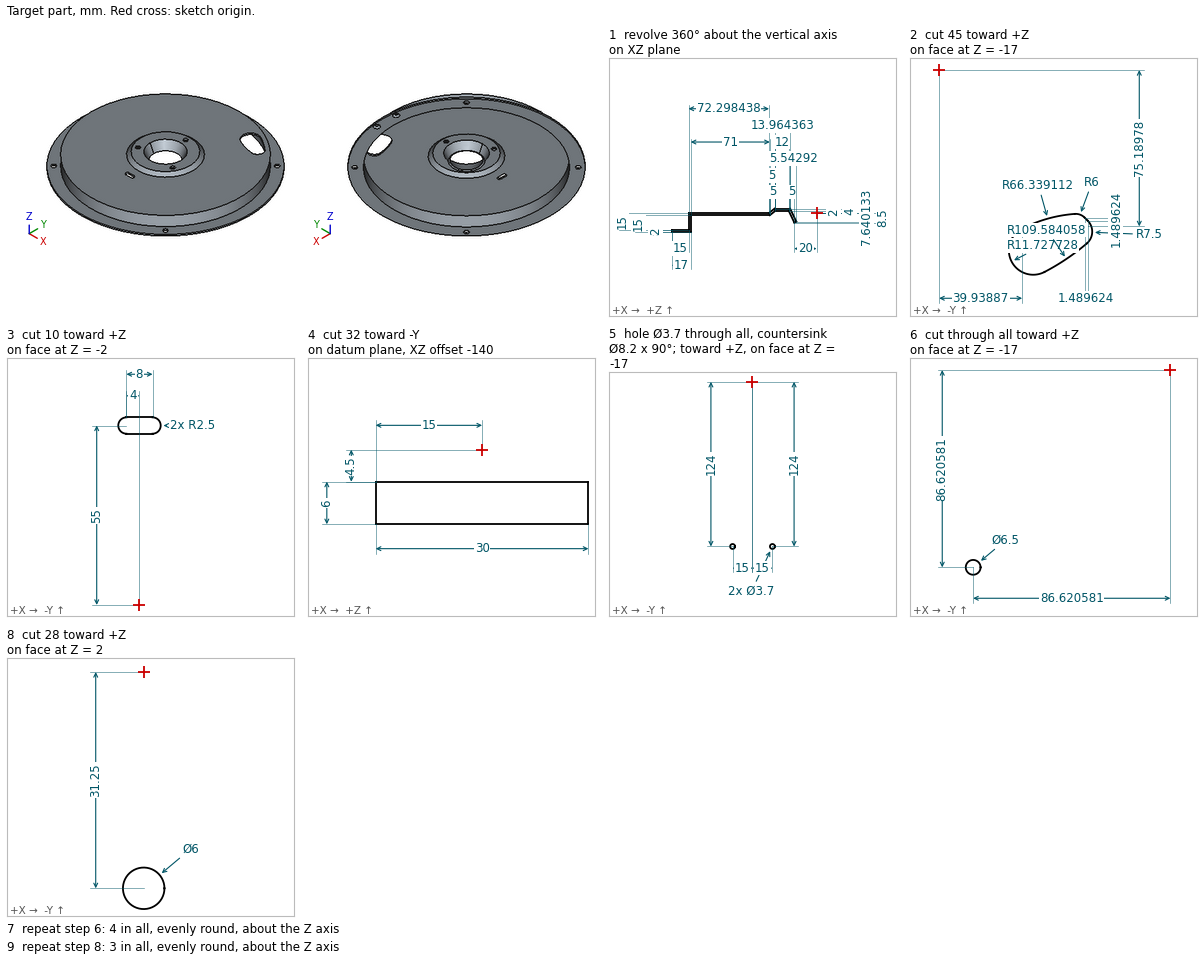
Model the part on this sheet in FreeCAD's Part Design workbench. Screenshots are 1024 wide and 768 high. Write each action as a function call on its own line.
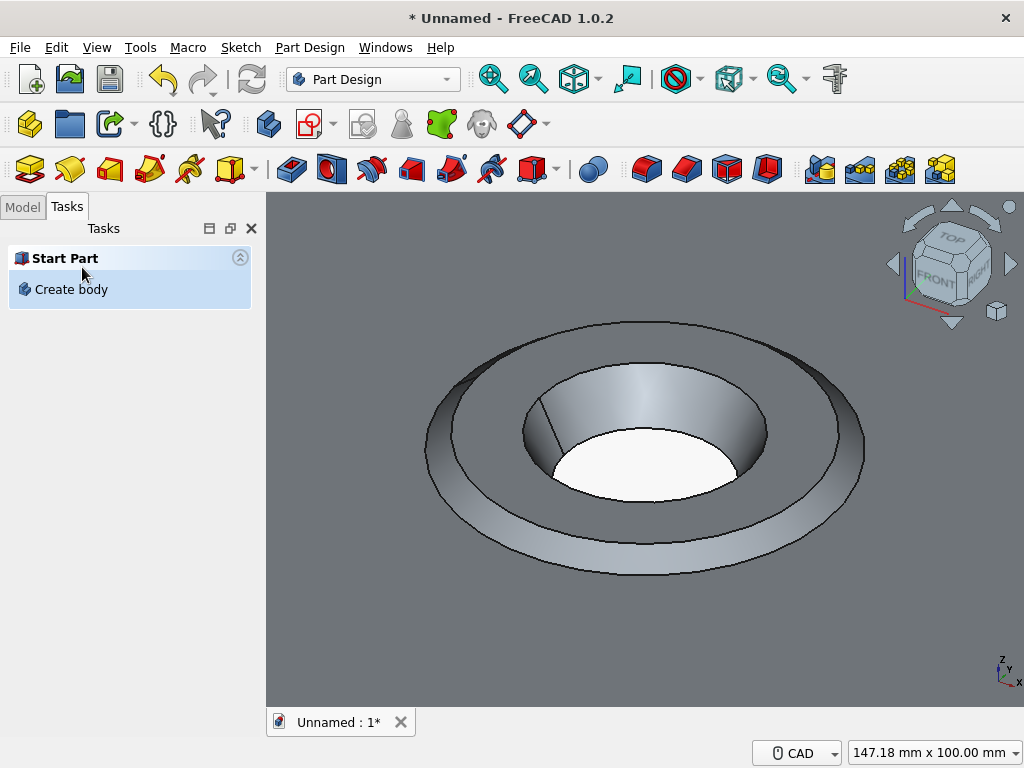
click(494, 80)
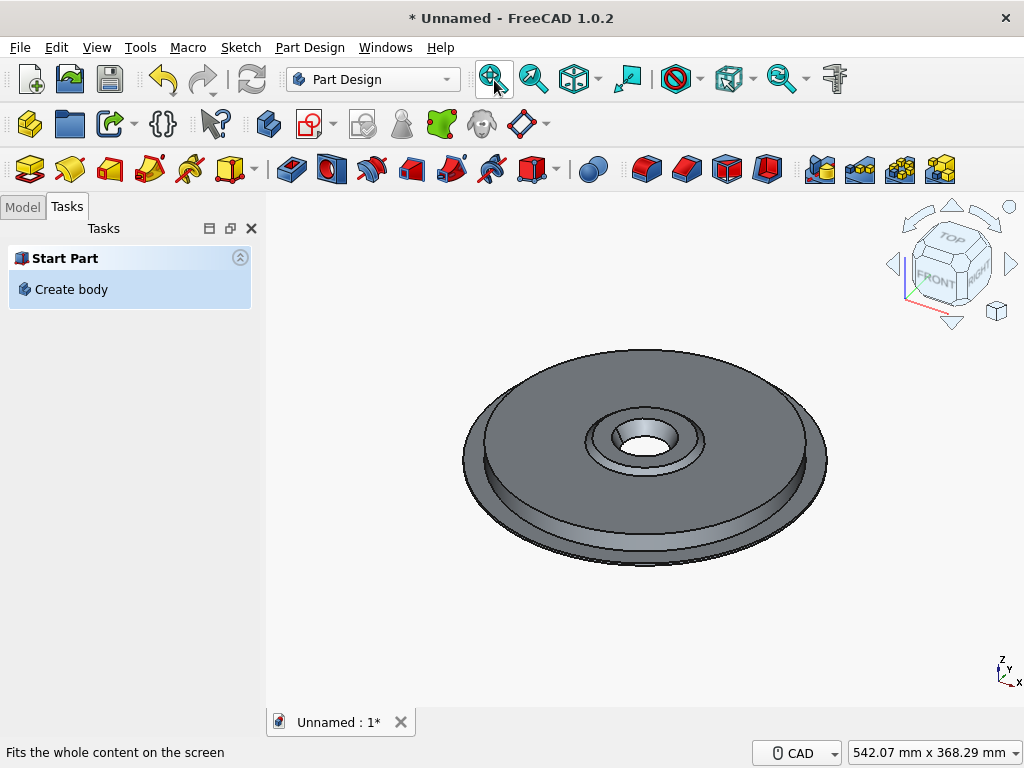
key(5)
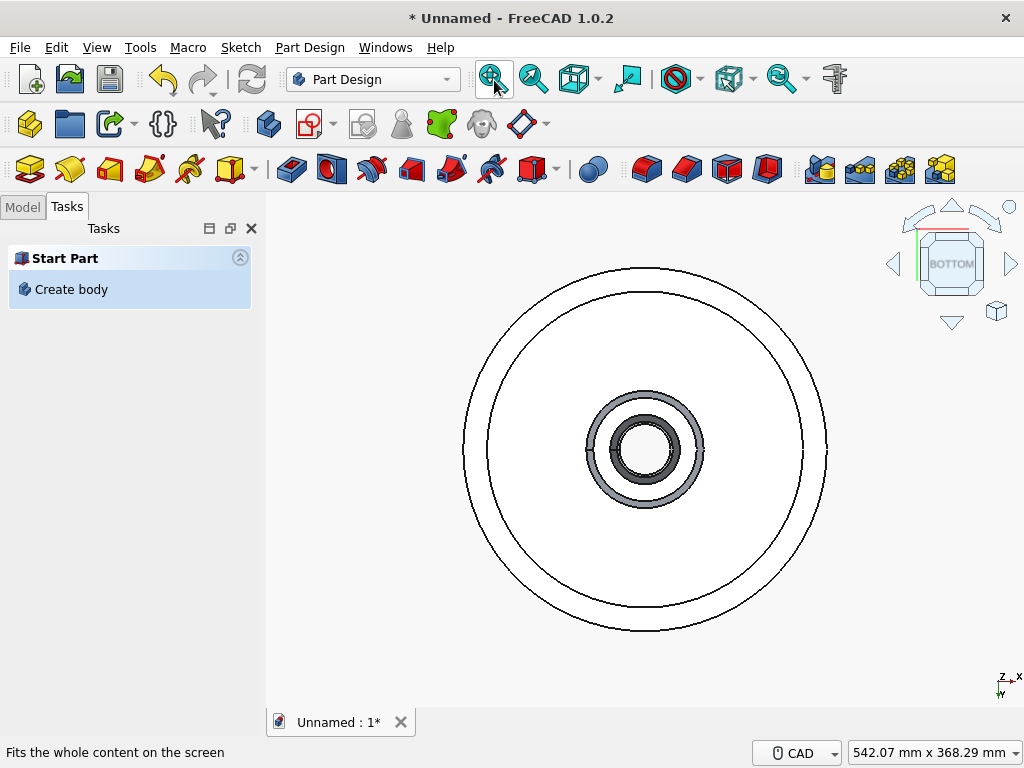
click(593, 293)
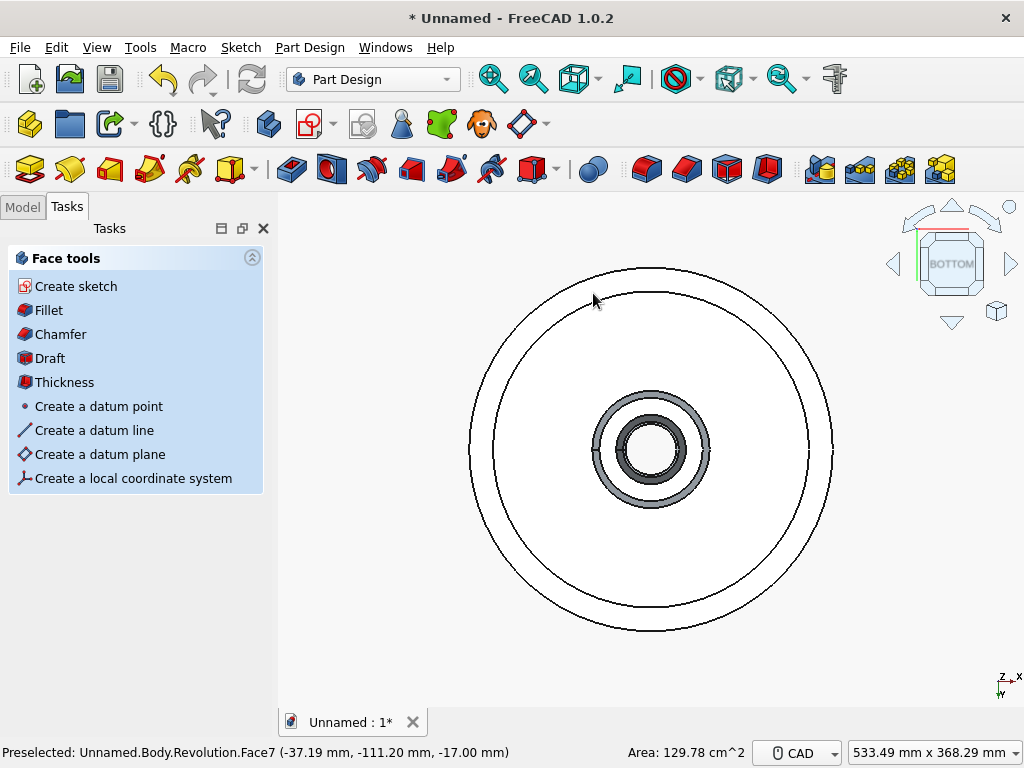
click(310, 124)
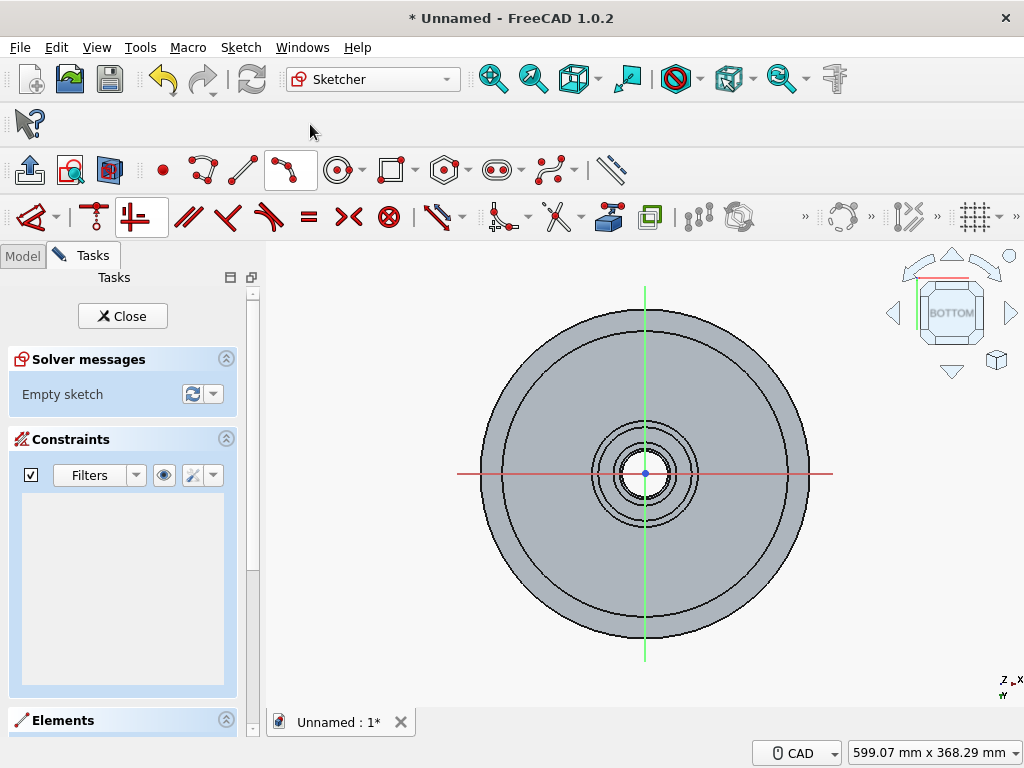
scroll(735, 596, up, 10)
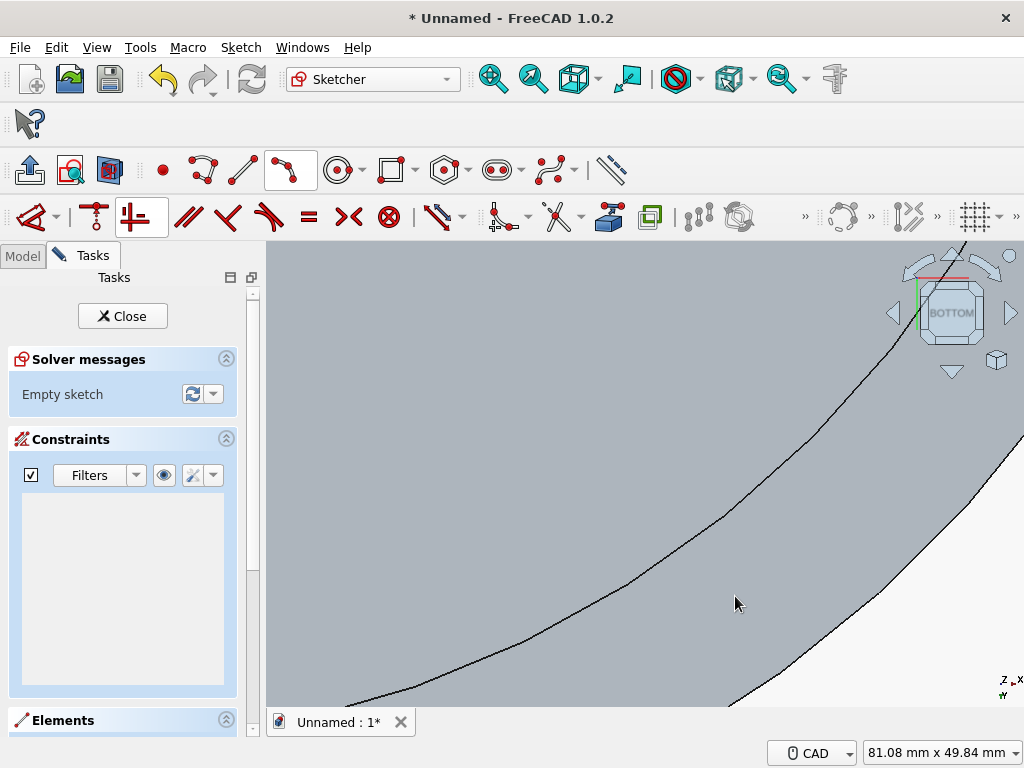
click(244, 170)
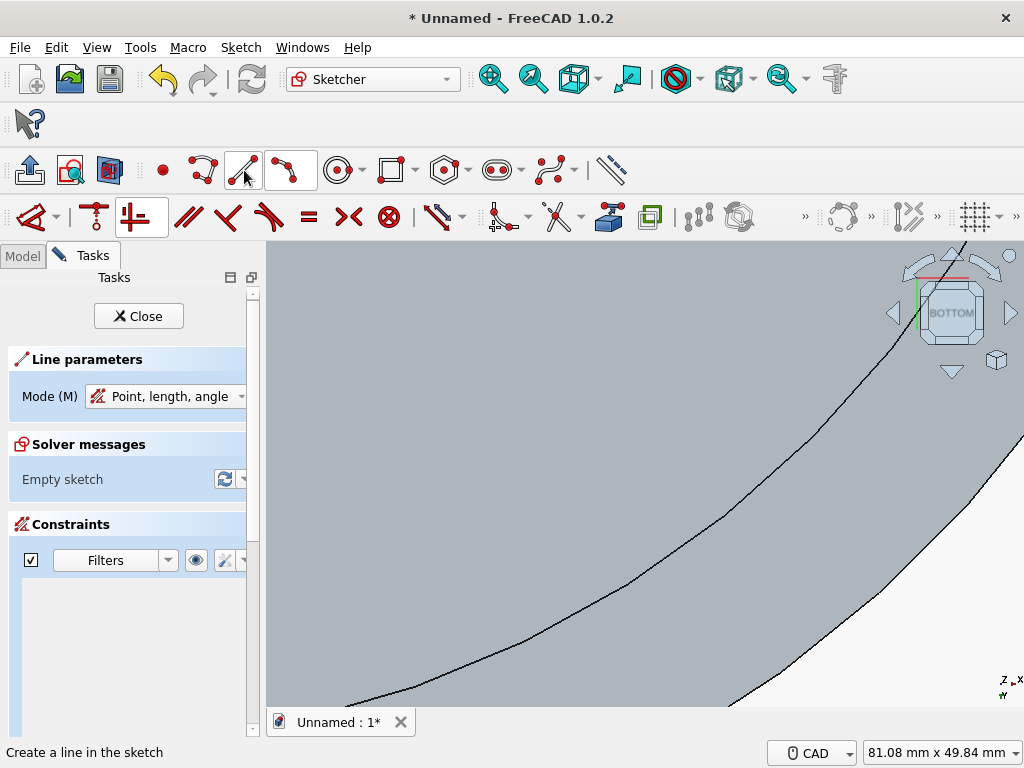
click(734, 367)
click(720, 353)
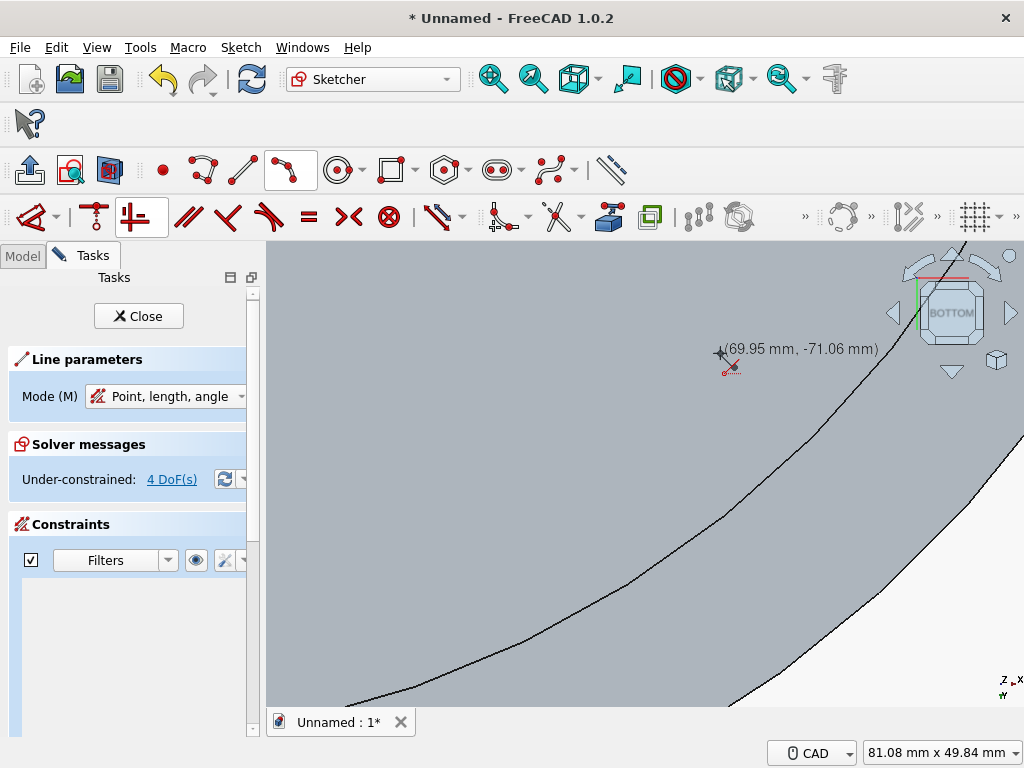
click(284, 170)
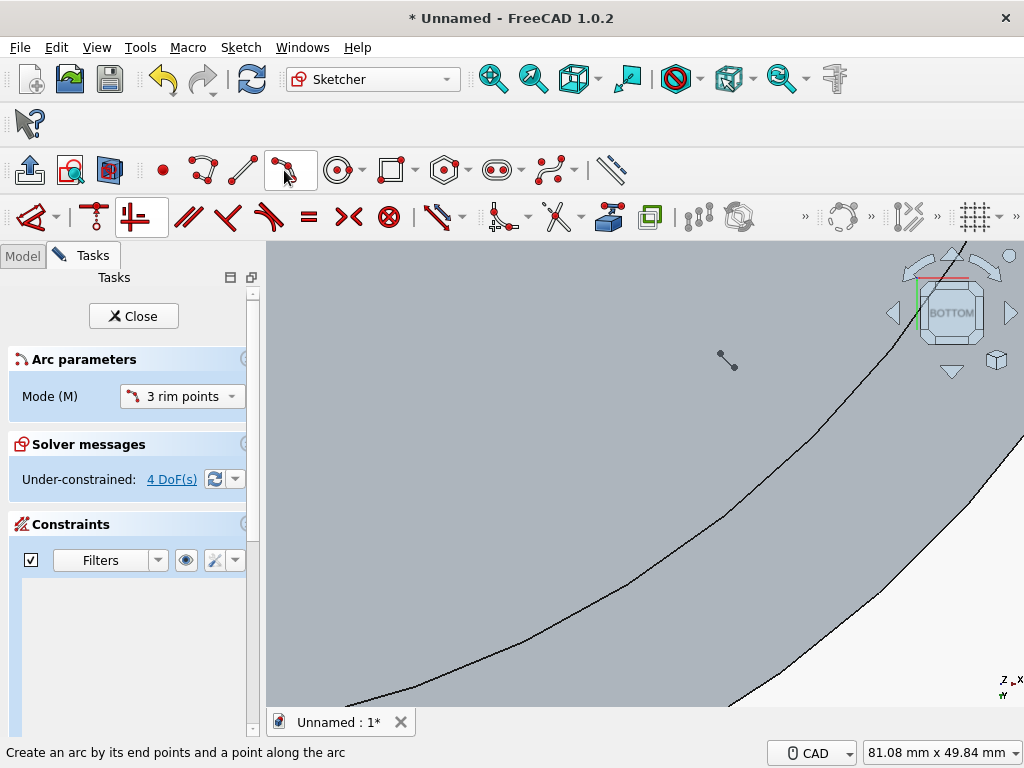
scroll(720, 353, up, 3)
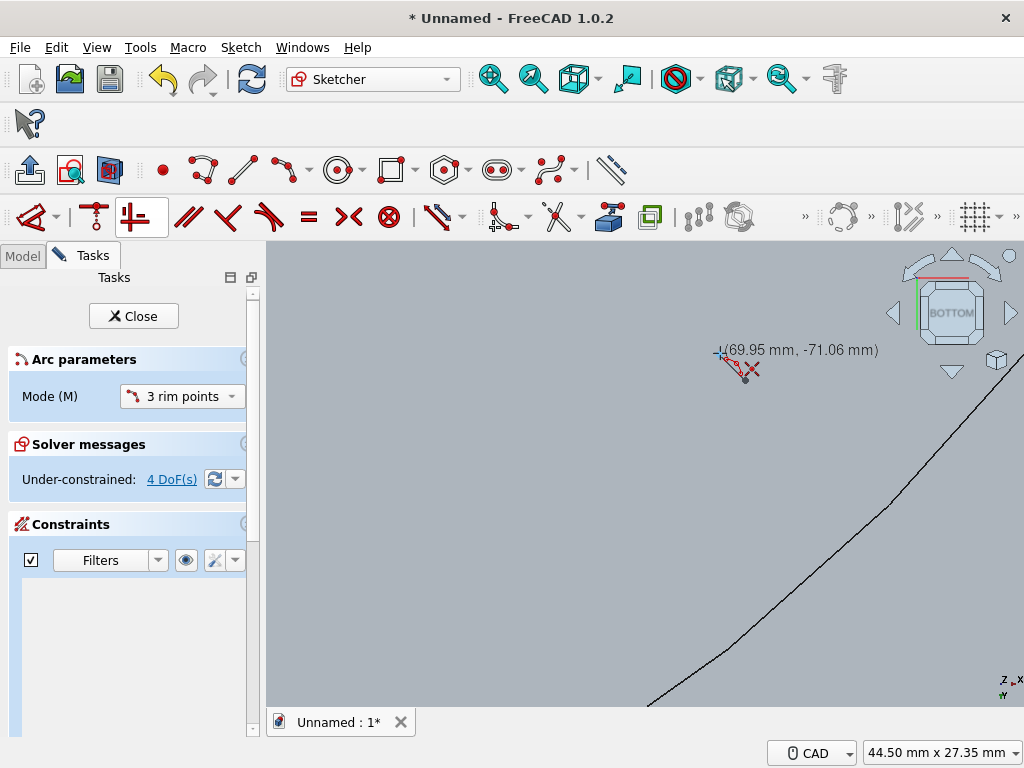
click(720, 355)
click(640, 323)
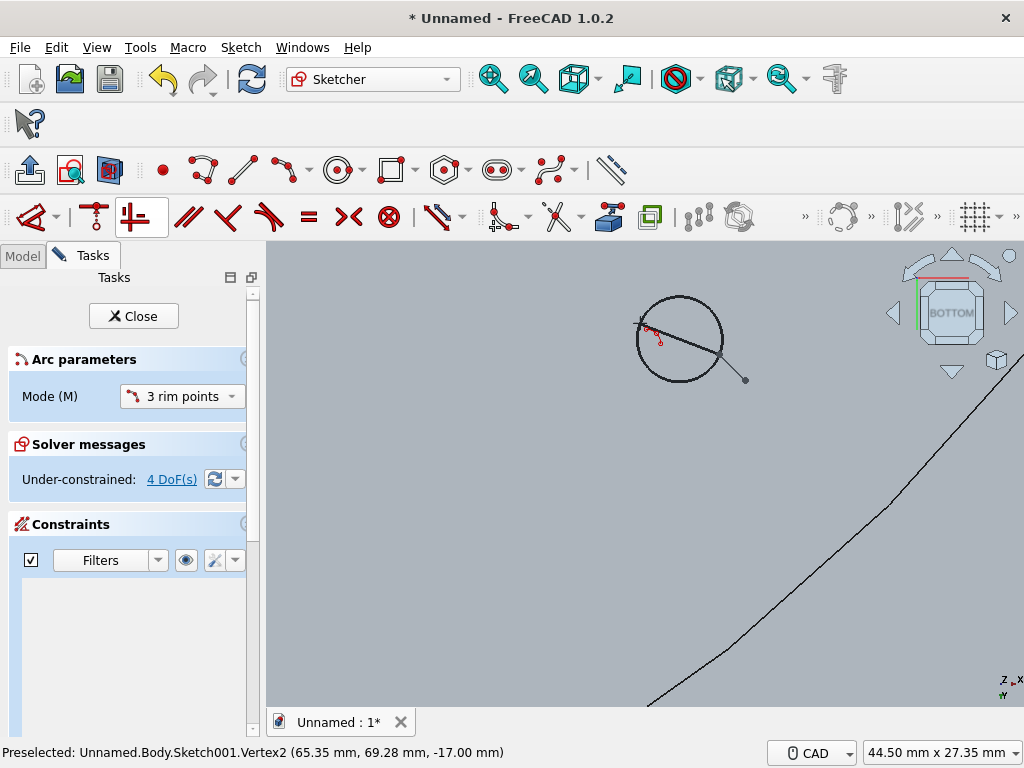
scroll(683, 329, up, 3)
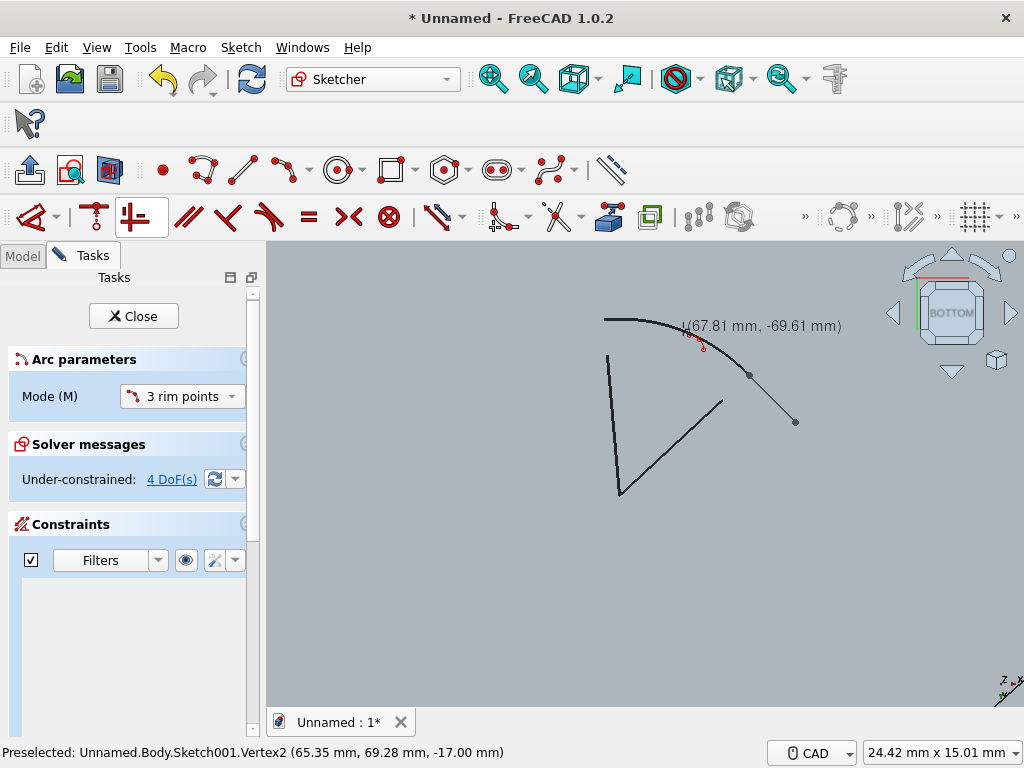
click(683, 329)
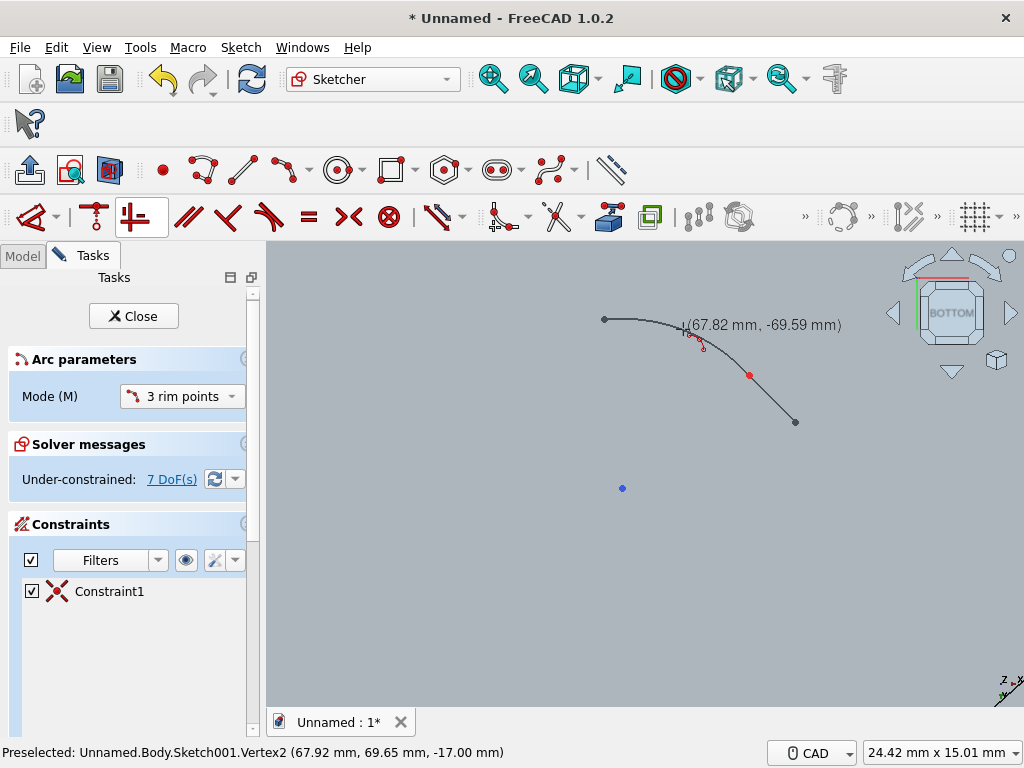
click(604, 320)